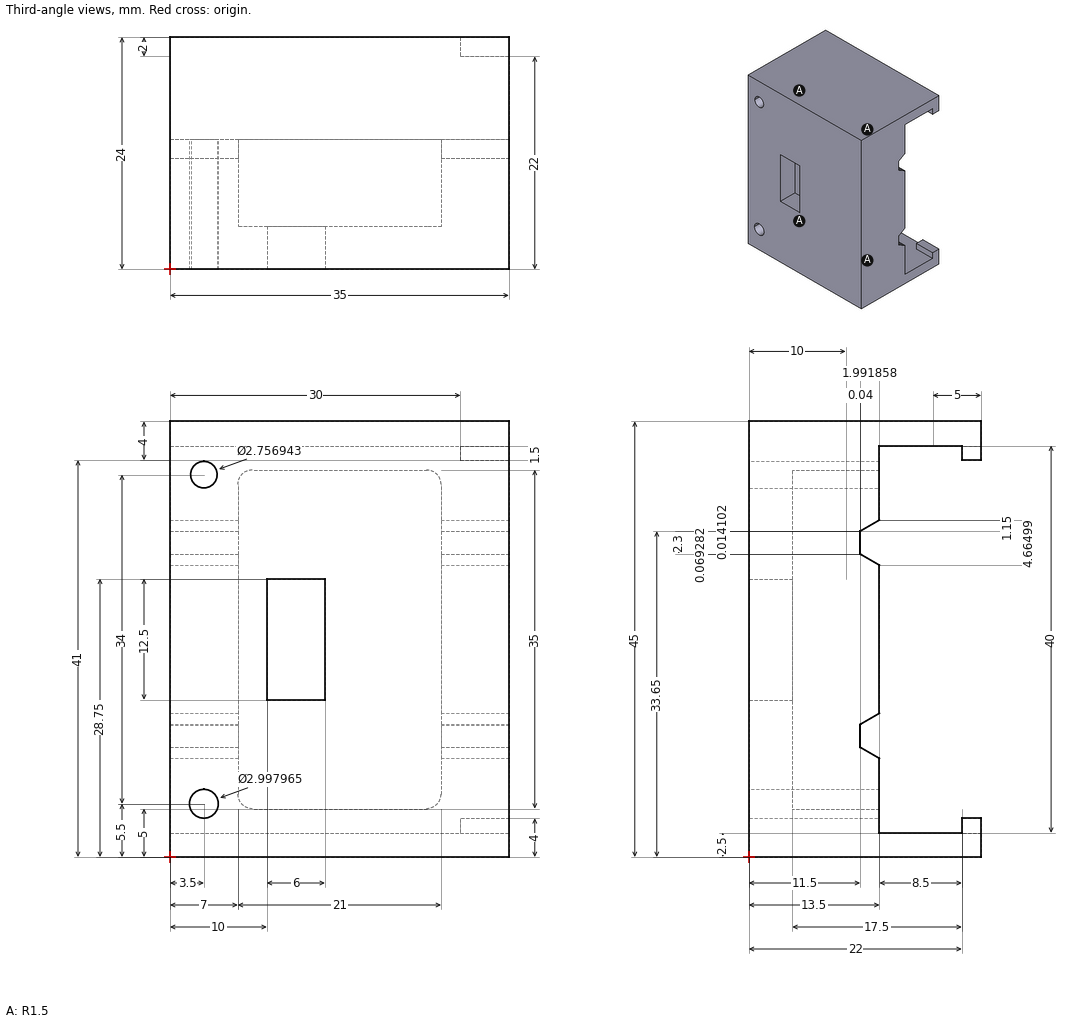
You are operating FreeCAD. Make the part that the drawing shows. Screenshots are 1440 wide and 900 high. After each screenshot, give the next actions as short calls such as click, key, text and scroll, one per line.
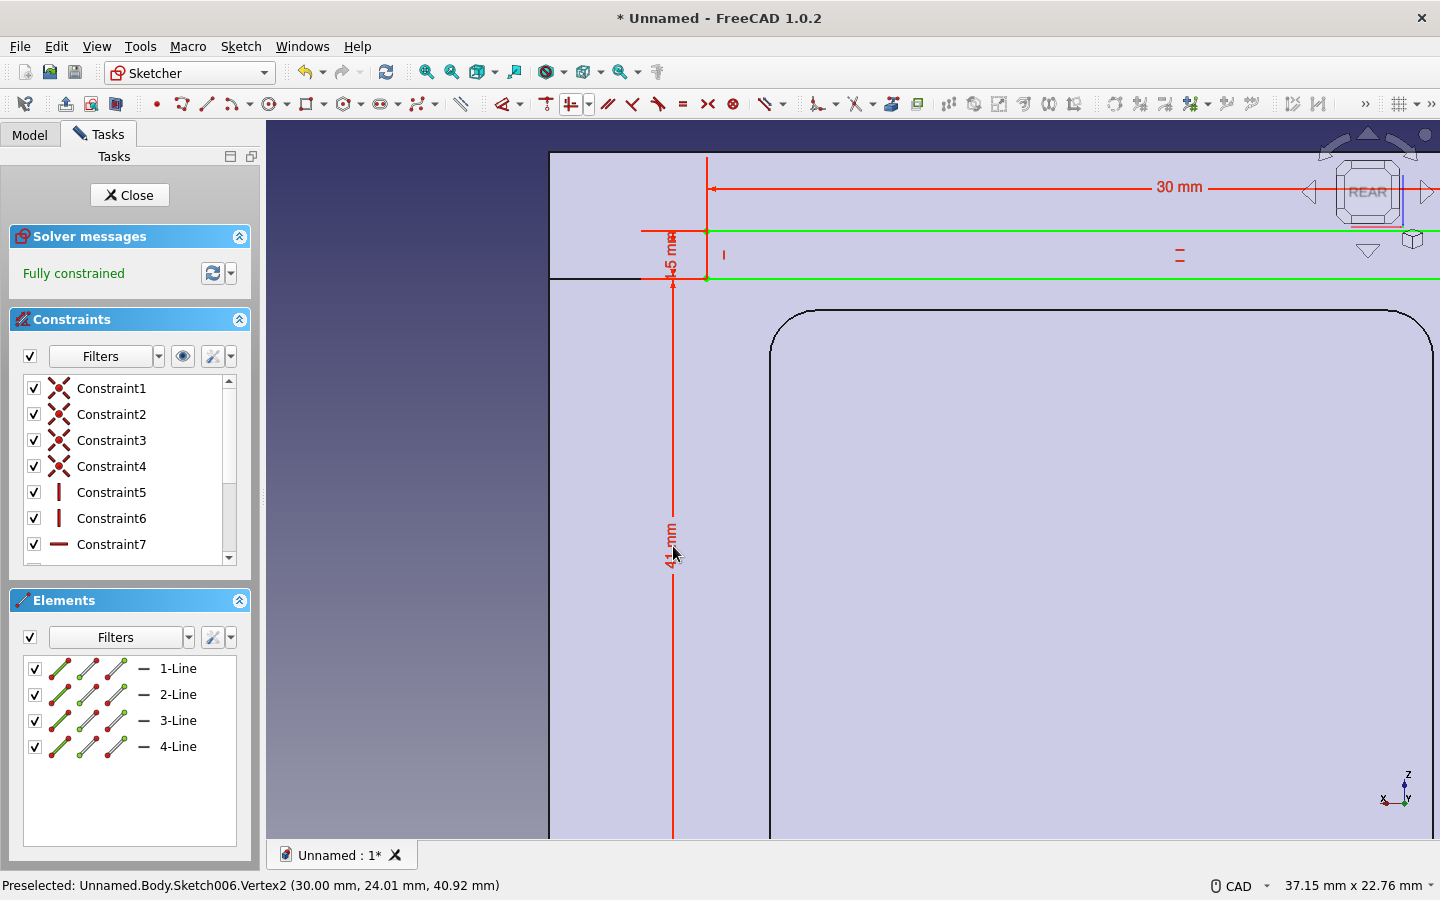
click(130, 195)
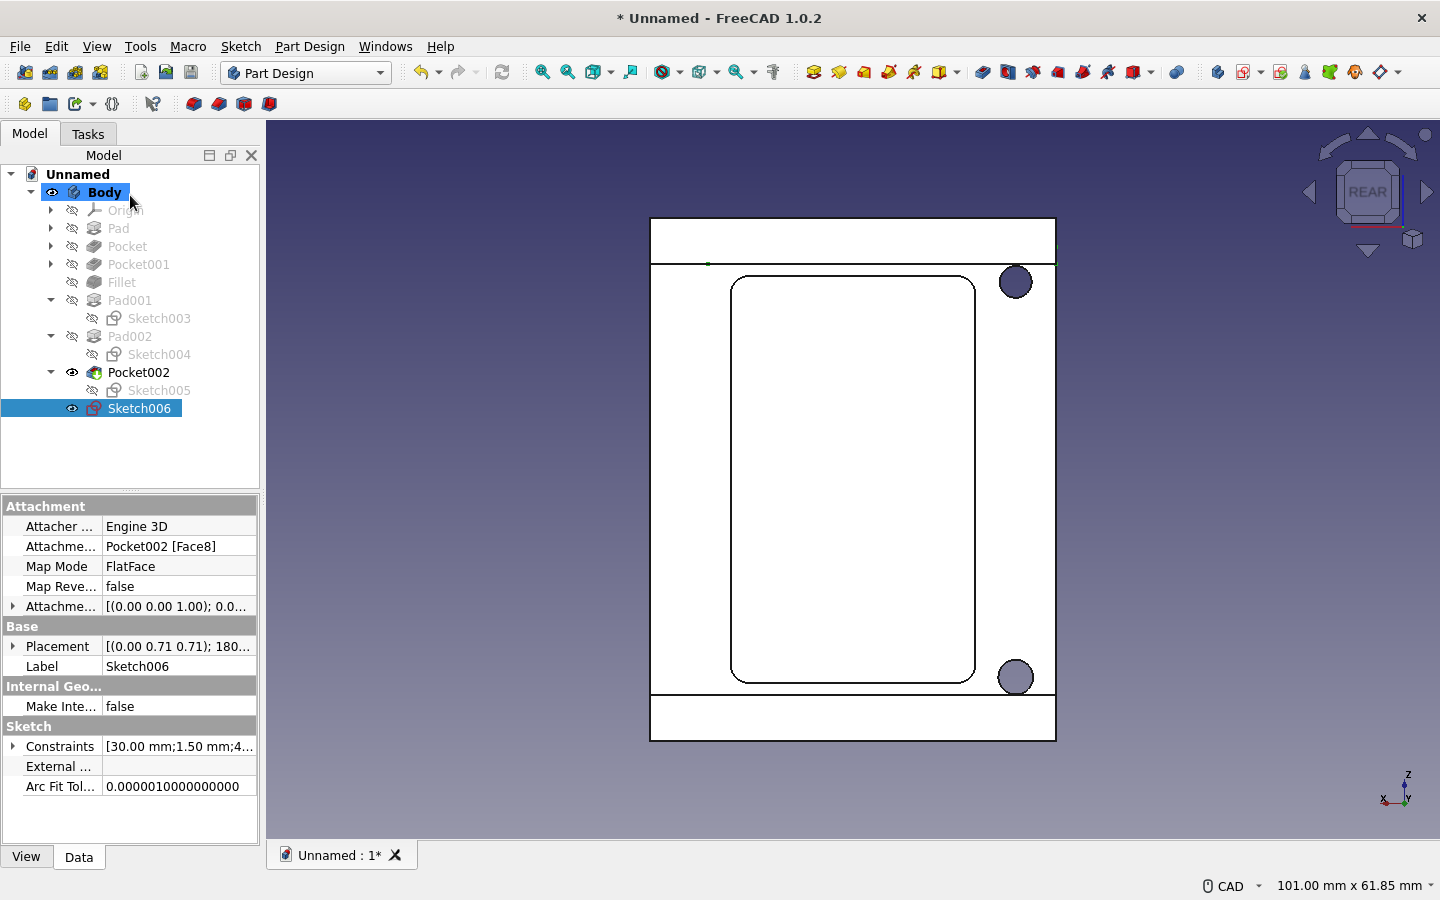
click(983, 72)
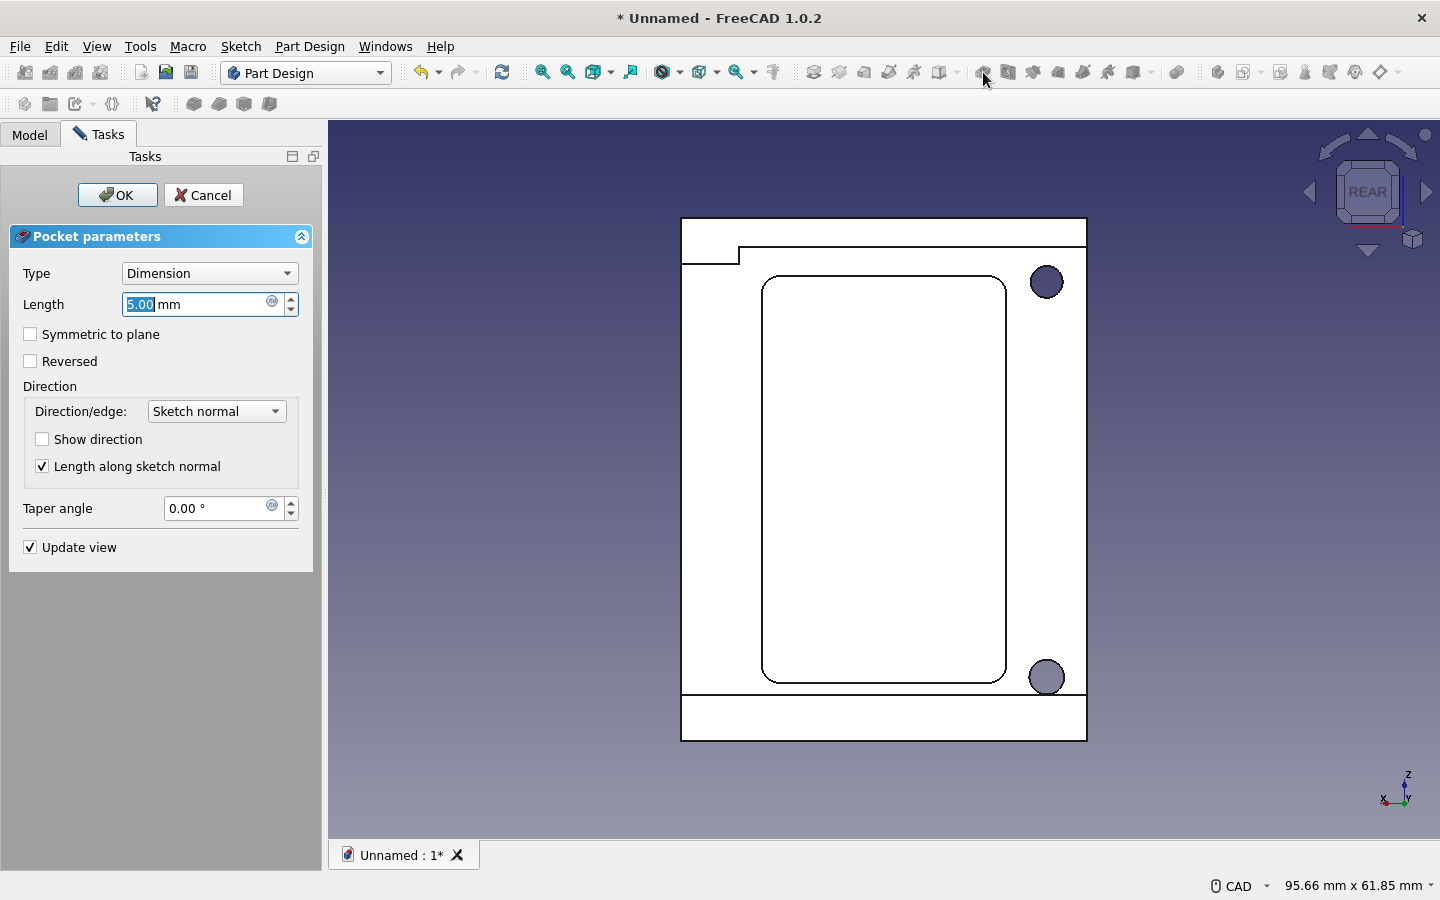
text(5)
key(Tab)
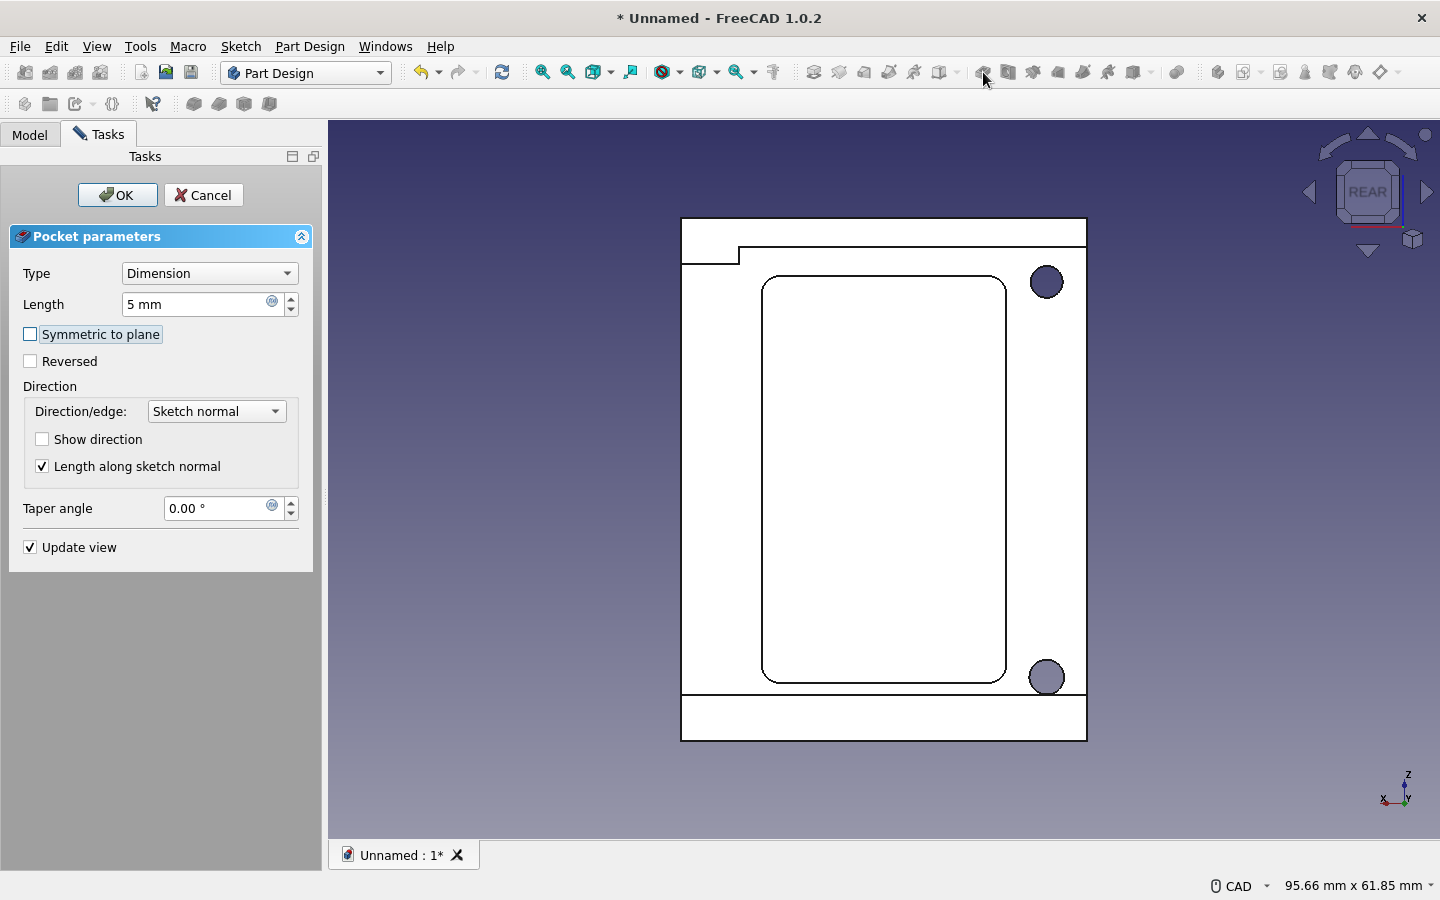
click(118, 195)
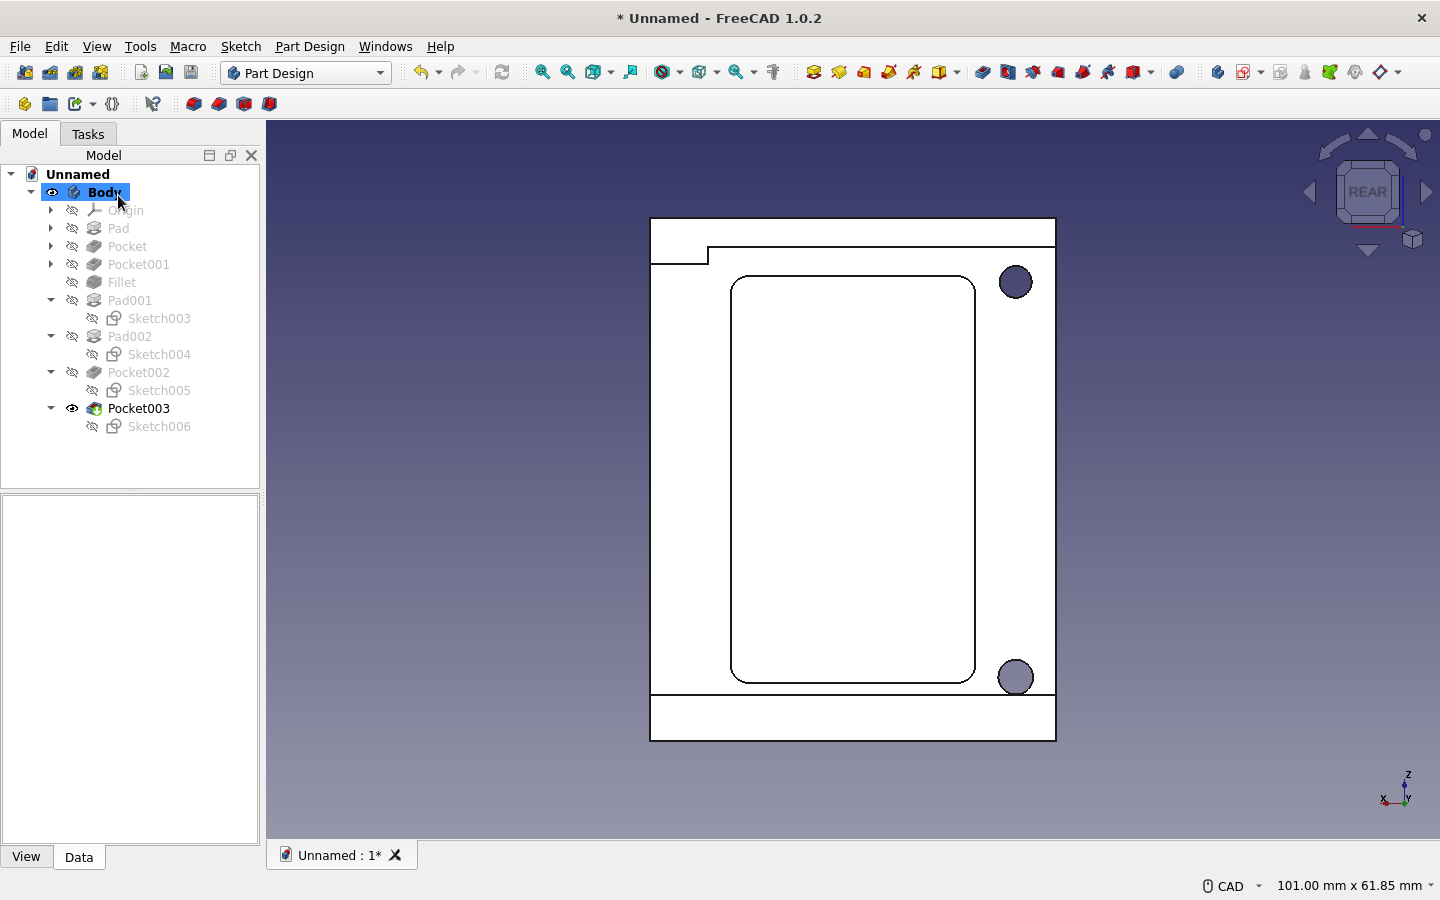
click(51, 210)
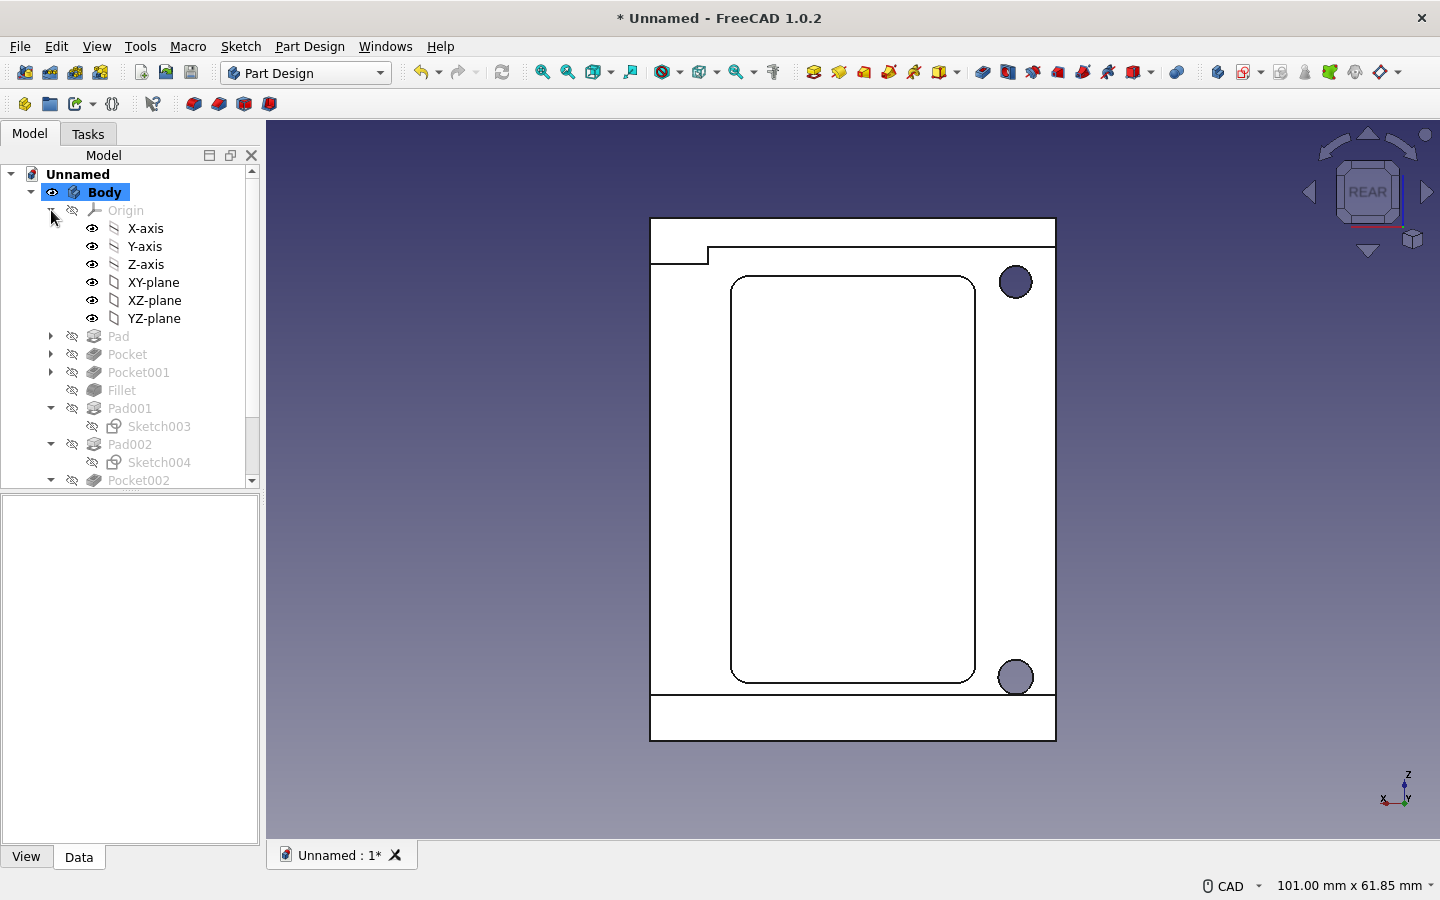
click(137, 282)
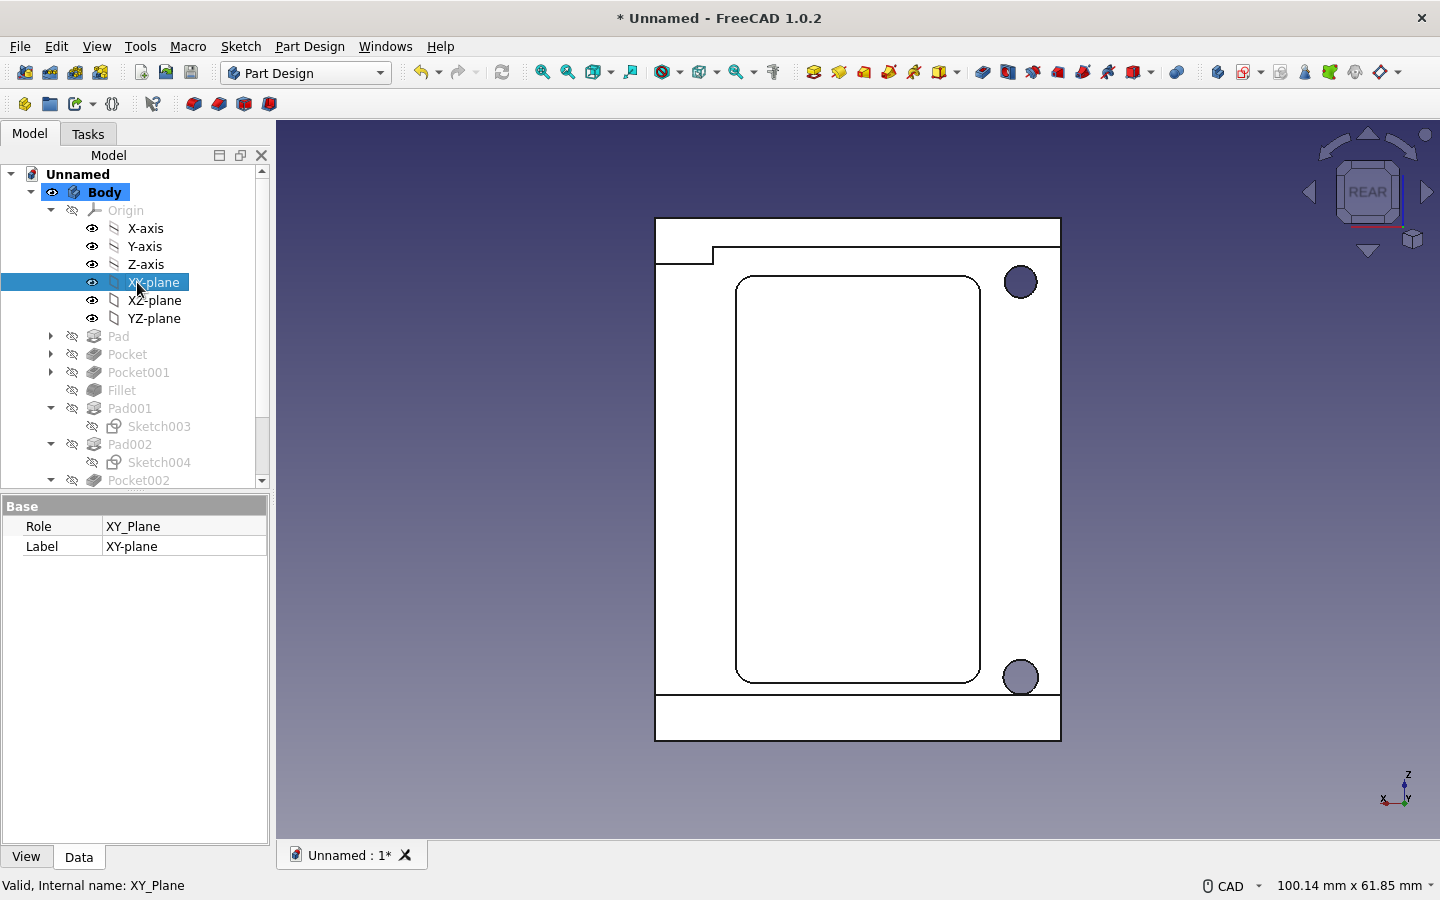
click(1380, 72)